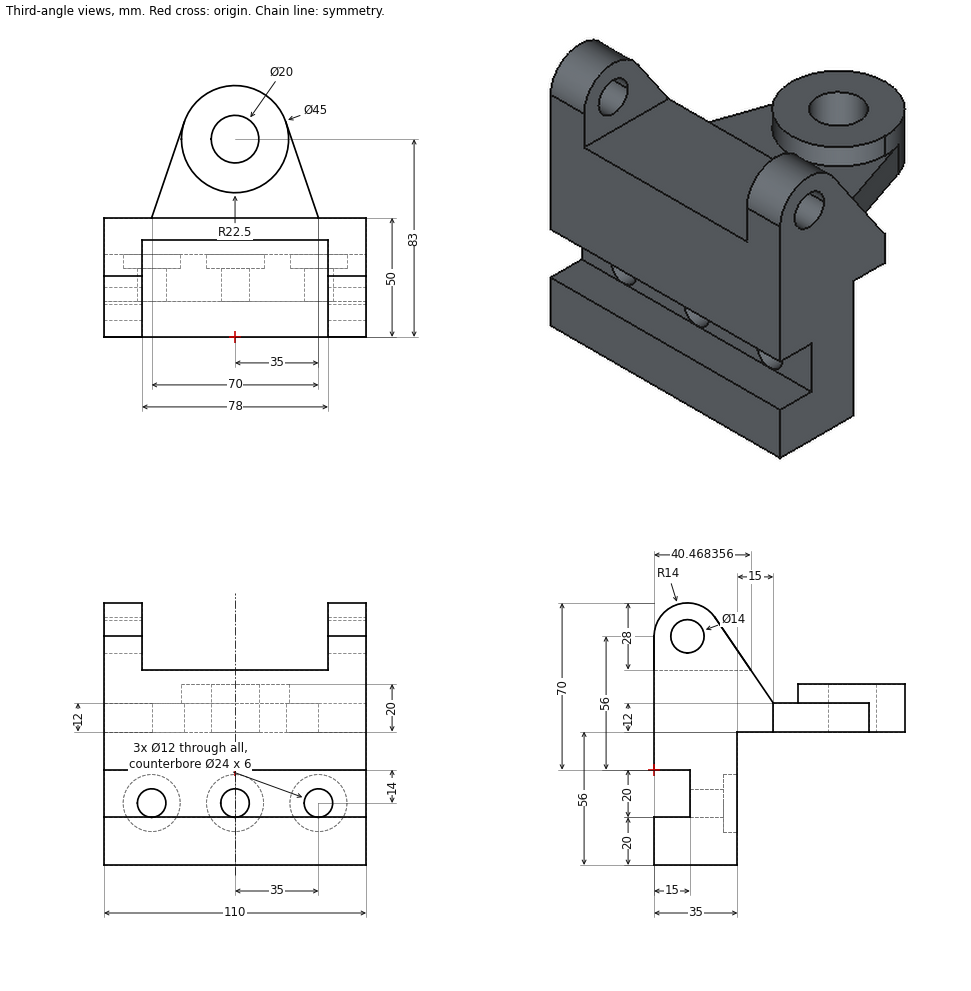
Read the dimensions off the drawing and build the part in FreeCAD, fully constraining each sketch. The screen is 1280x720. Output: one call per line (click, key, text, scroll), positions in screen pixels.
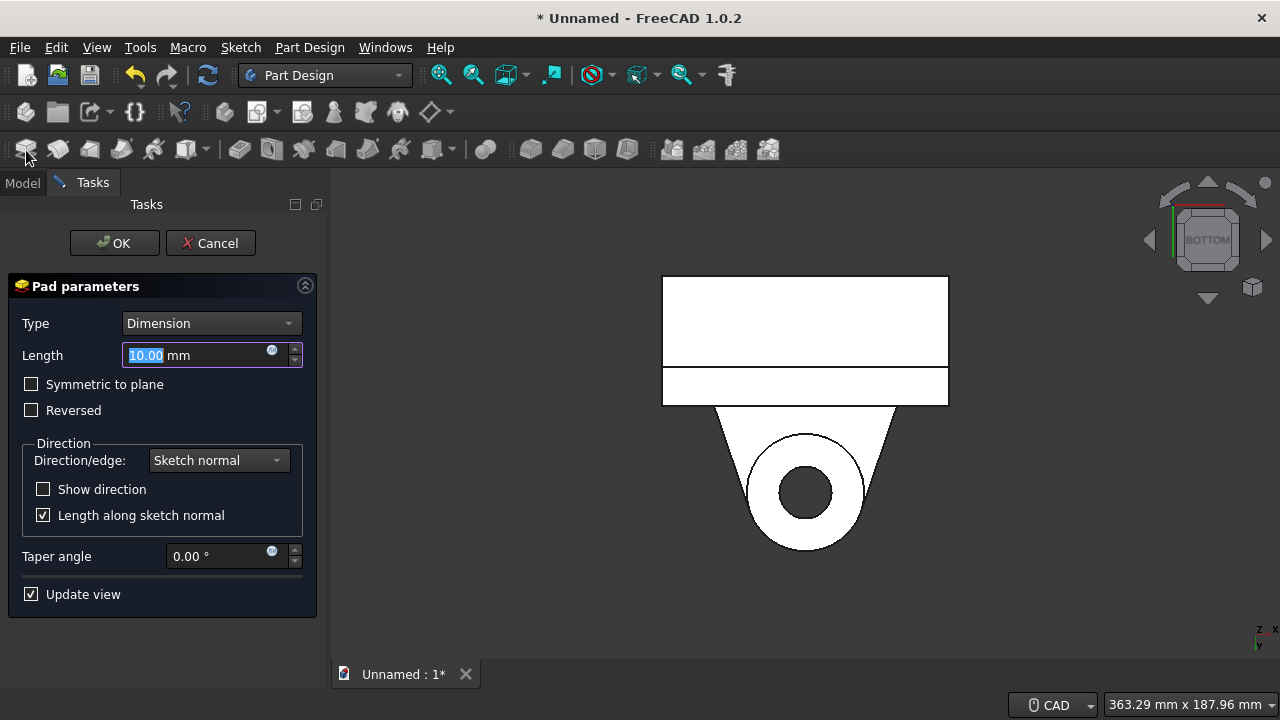
text(12)
key(Tab)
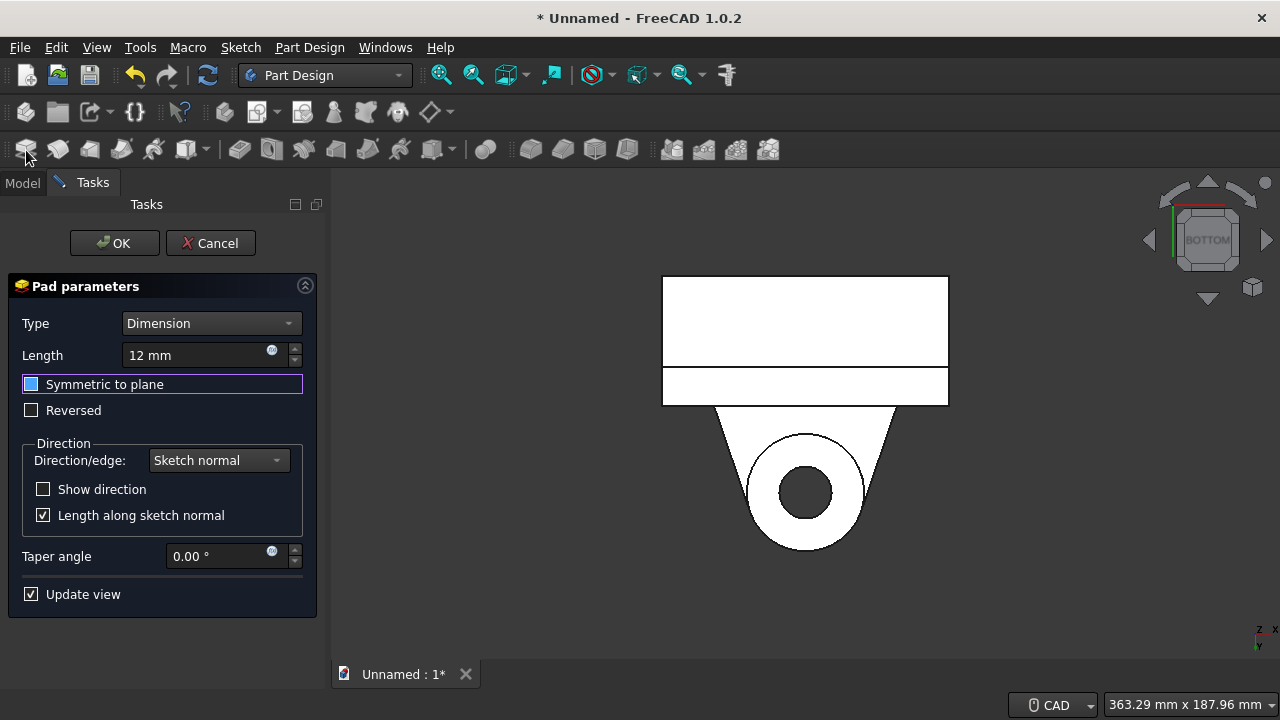
click(30, 410)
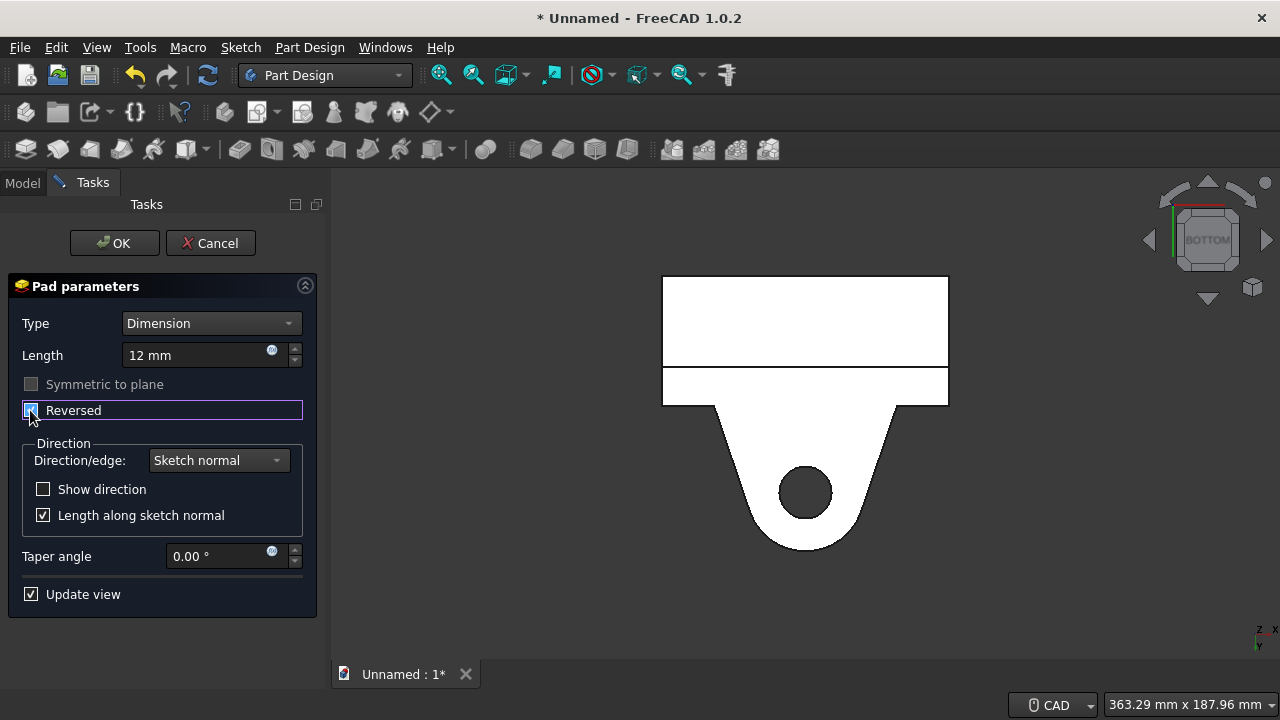
click(115, 243)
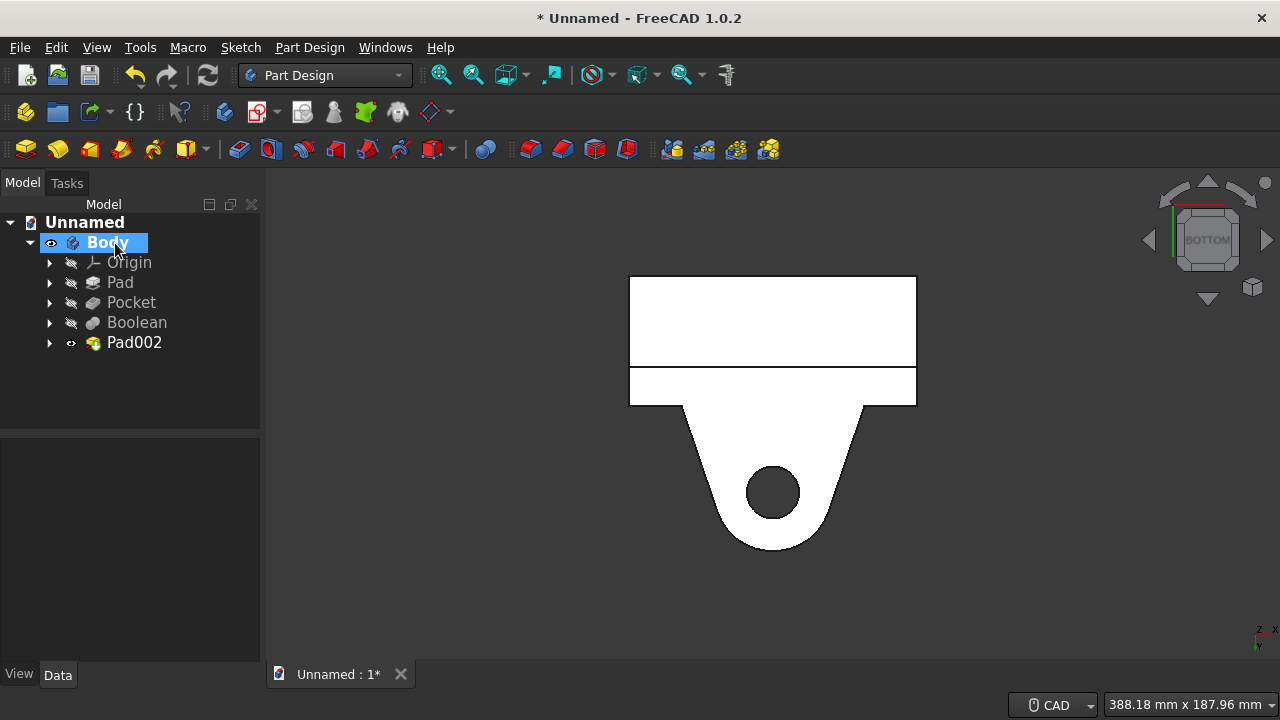
key(4)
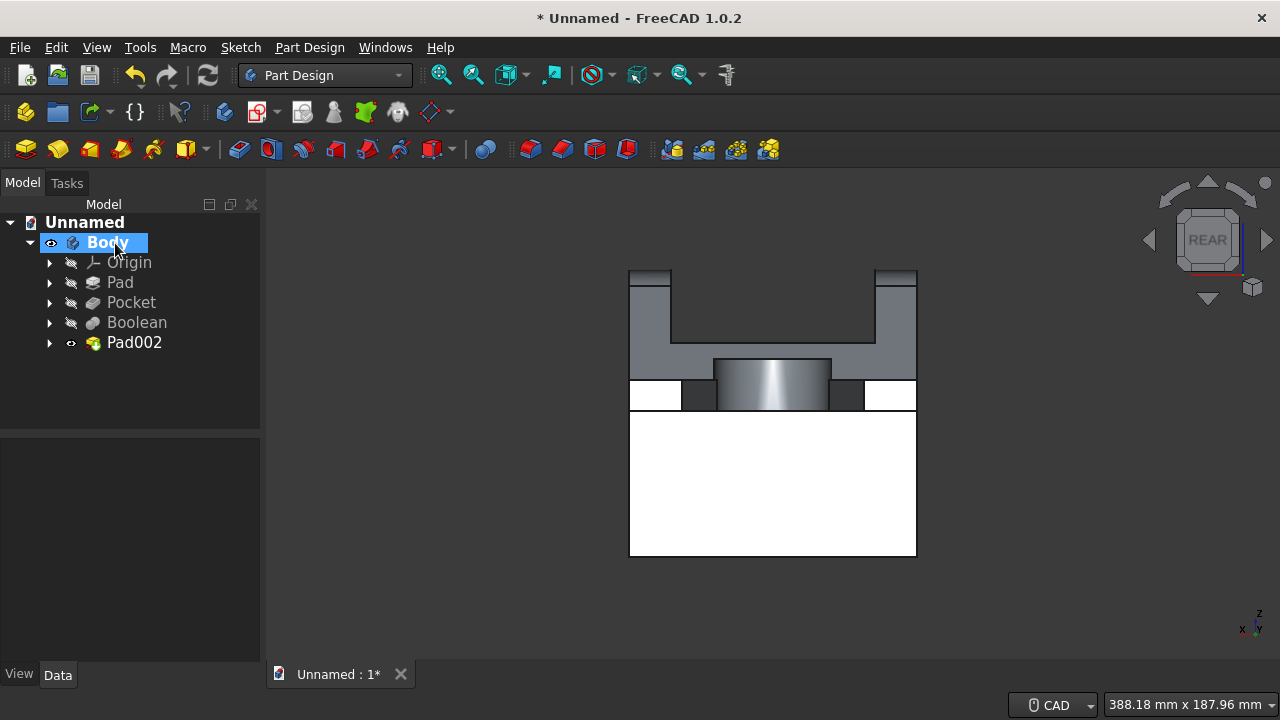
click(732, 483)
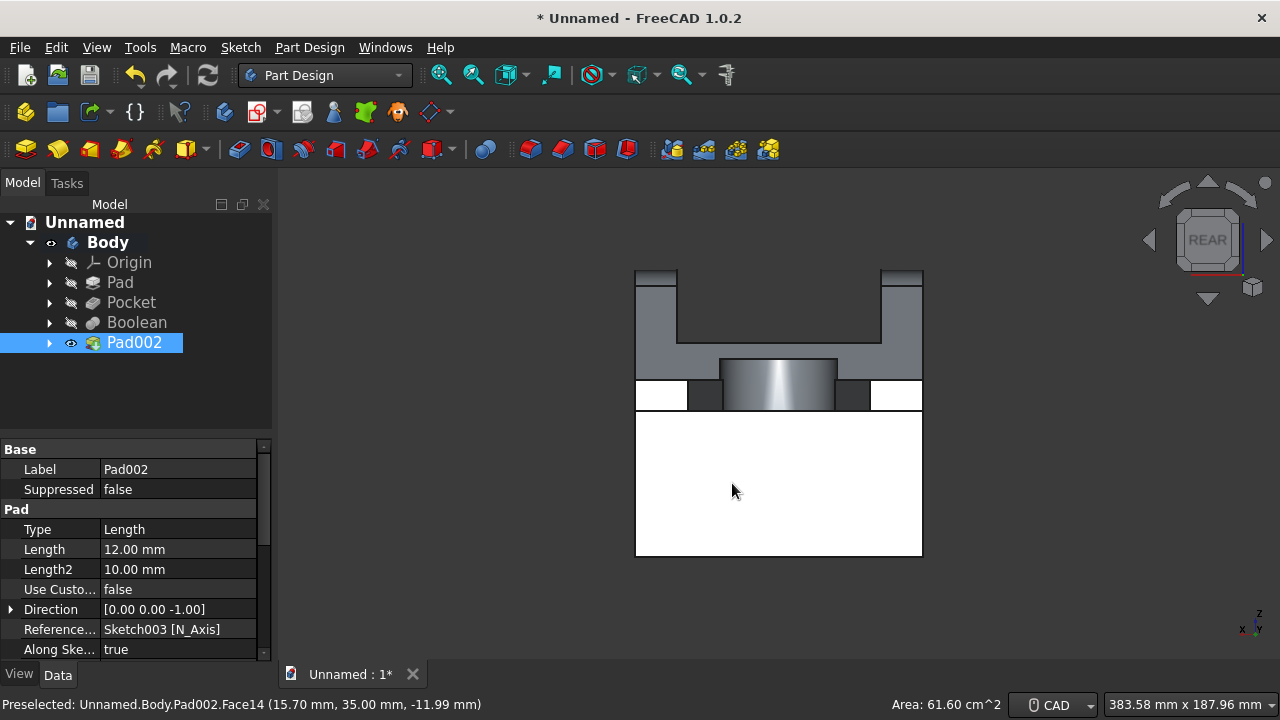
click(258, 112)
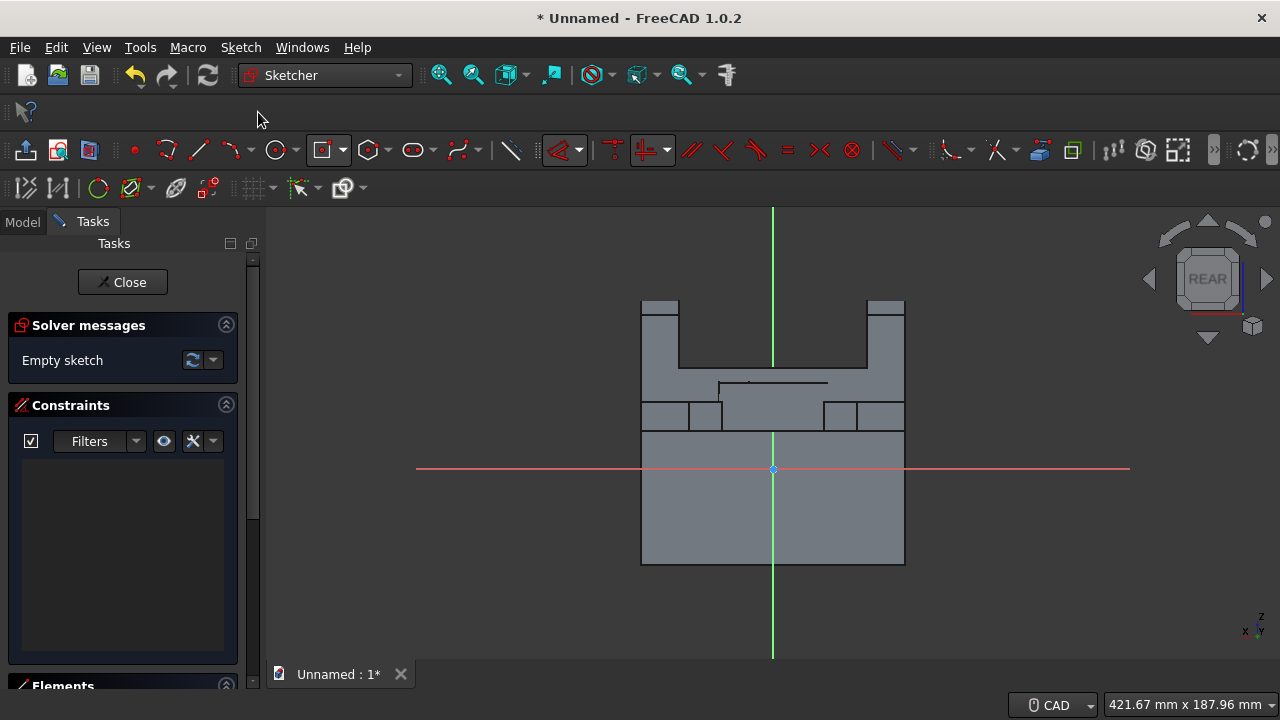
scroll(813, 528, up, 5)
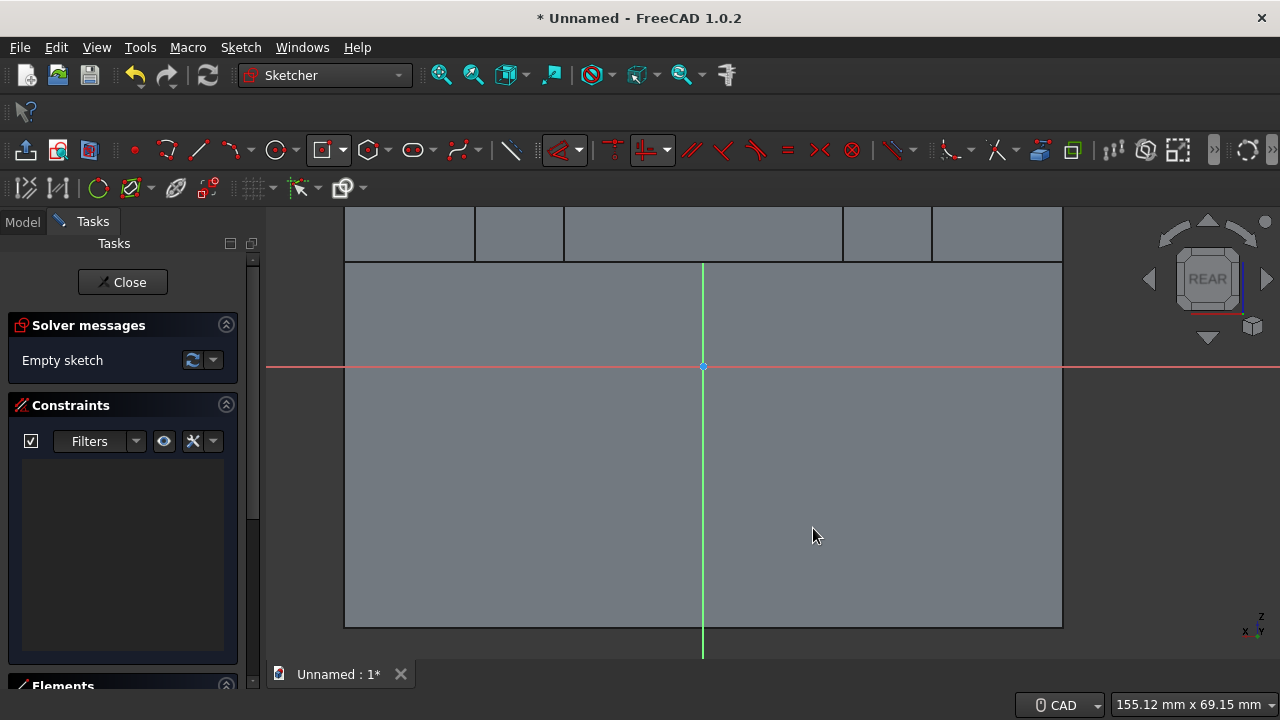
key(g)
key(c)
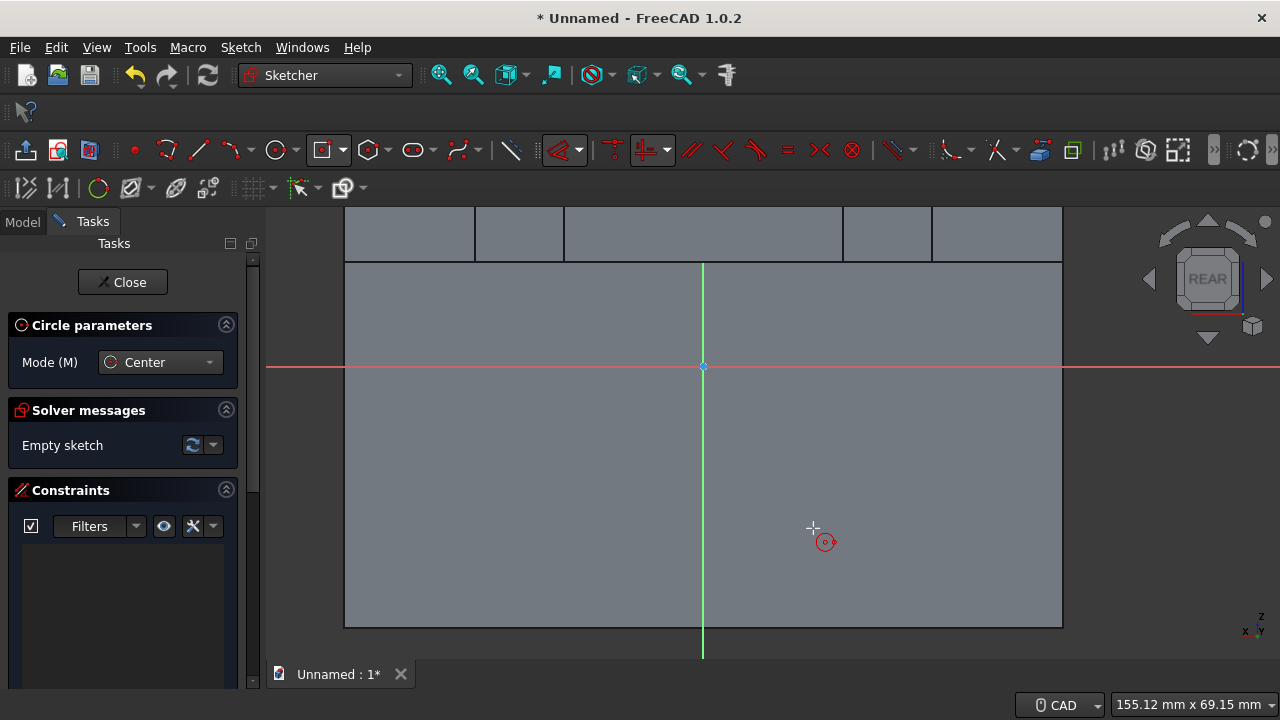
click(475, 458)
click(502, 430)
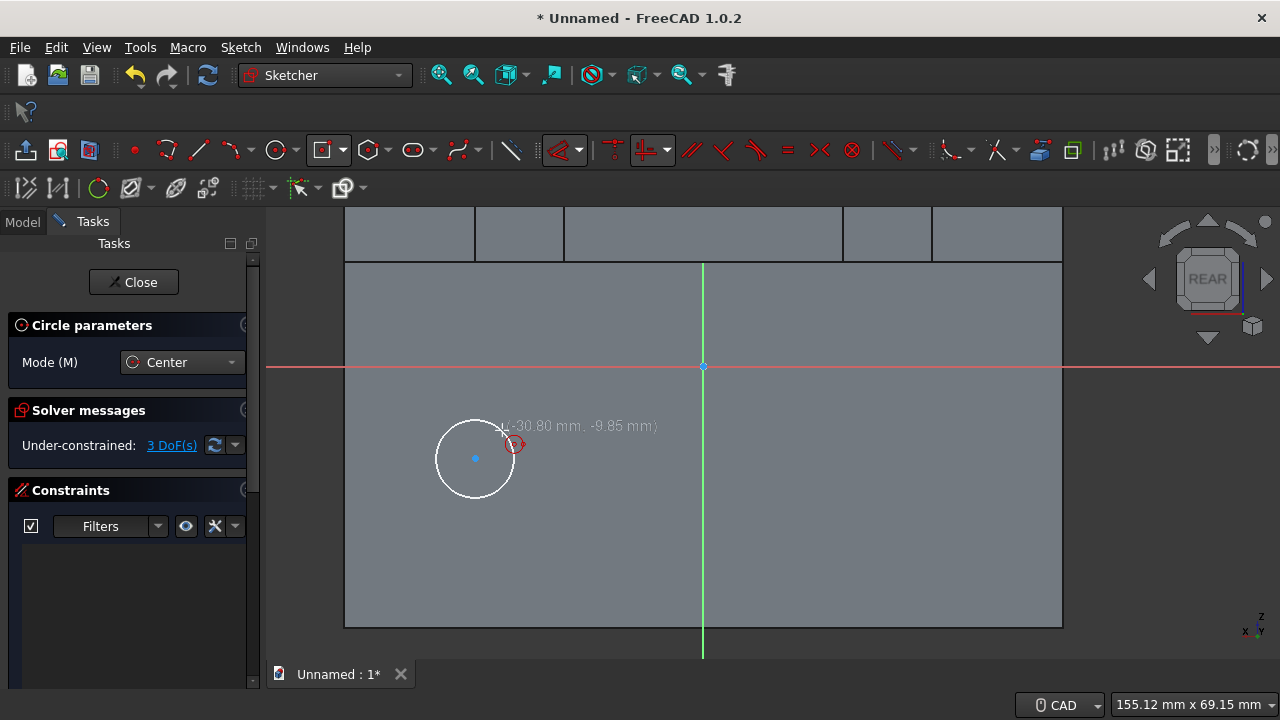
click(703, 458)
click(731, 430)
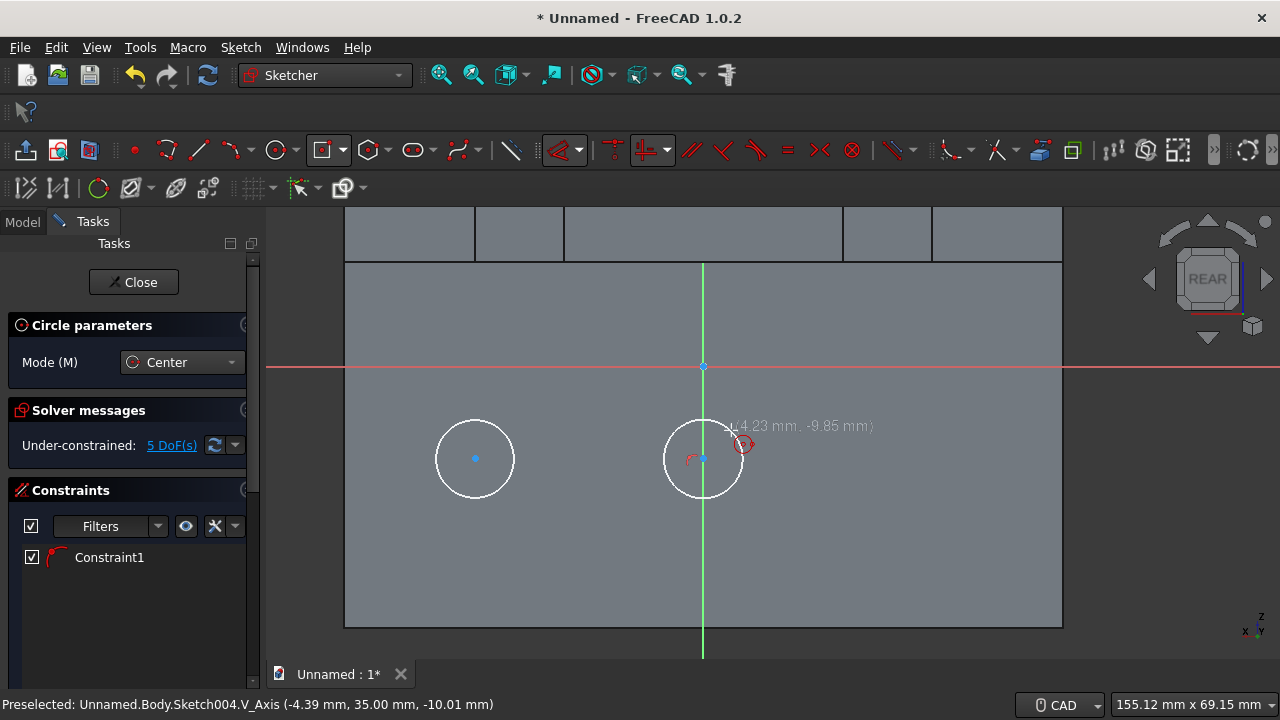
click(932, 458)
click(960, 430)
key(Escape)